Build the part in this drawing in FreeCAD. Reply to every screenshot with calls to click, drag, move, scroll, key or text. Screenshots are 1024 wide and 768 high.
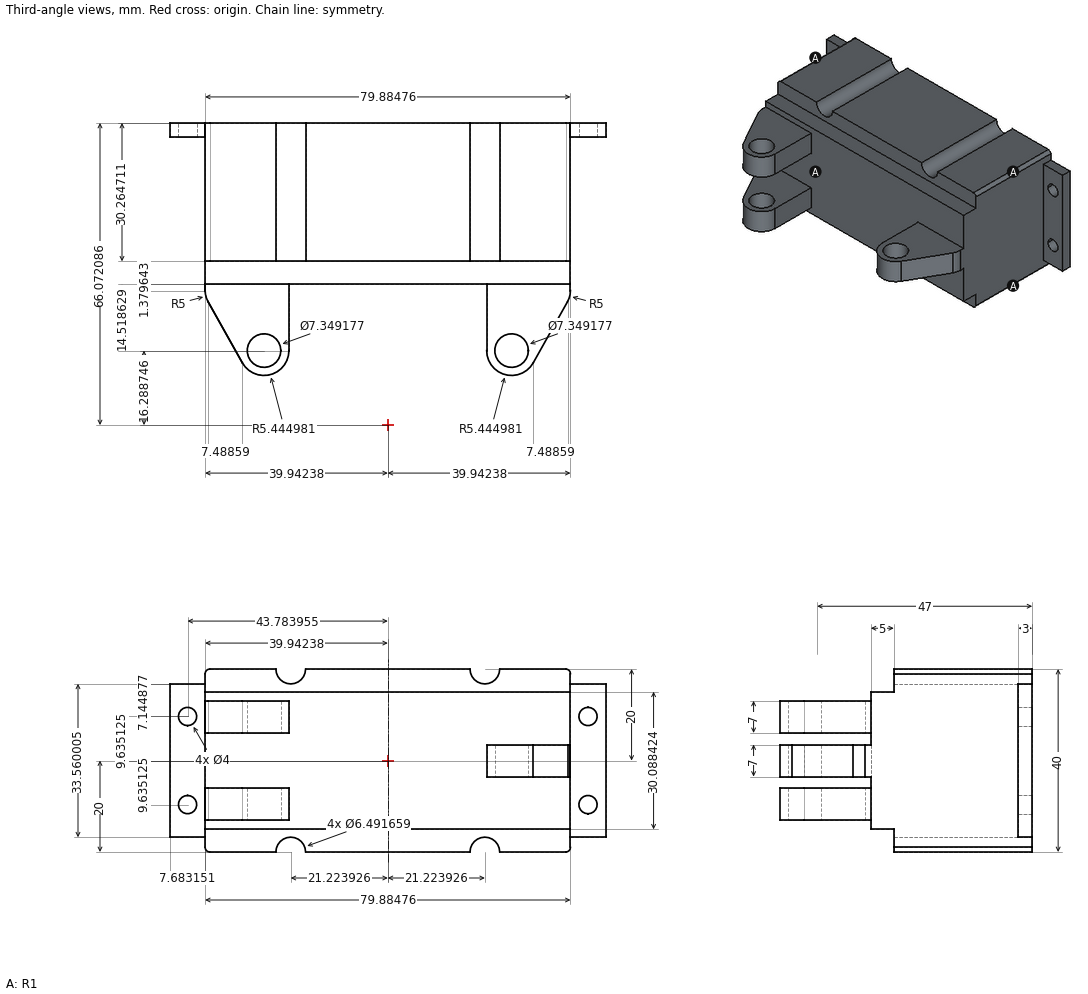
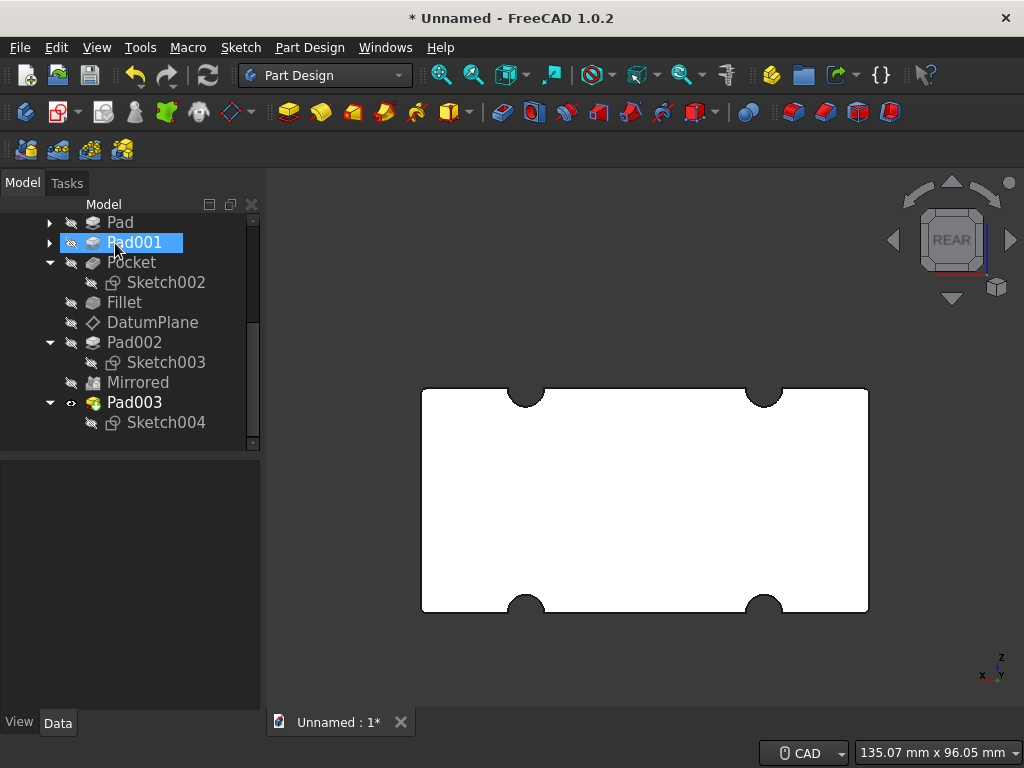
click(645, 500)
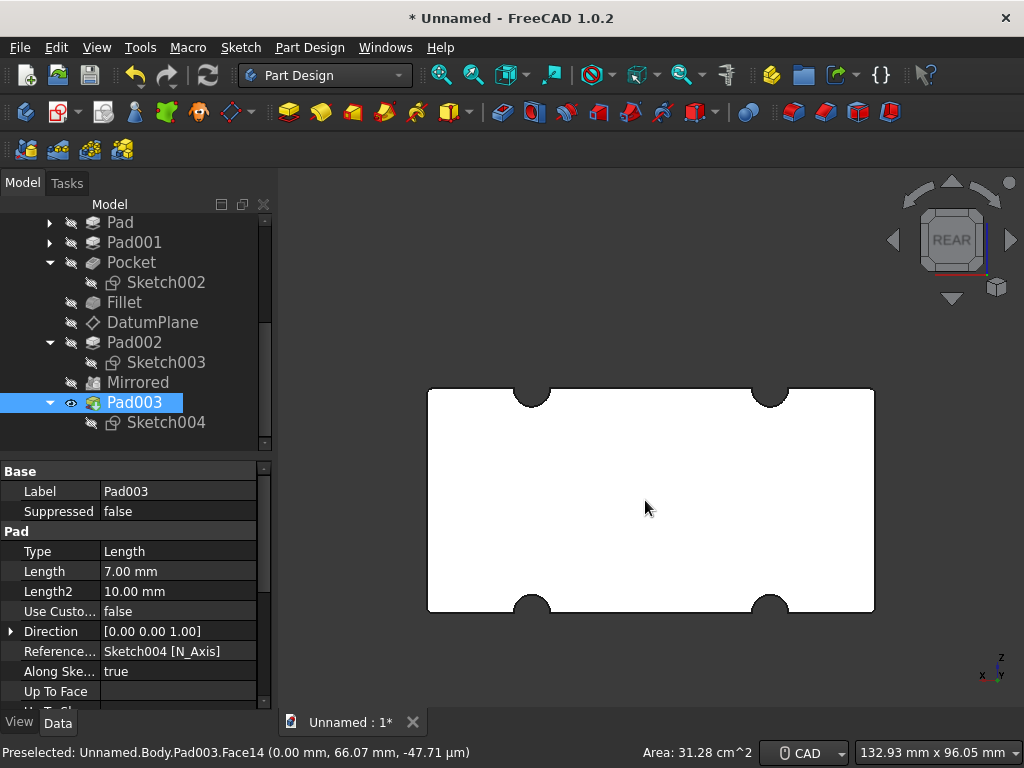
click(58, 112)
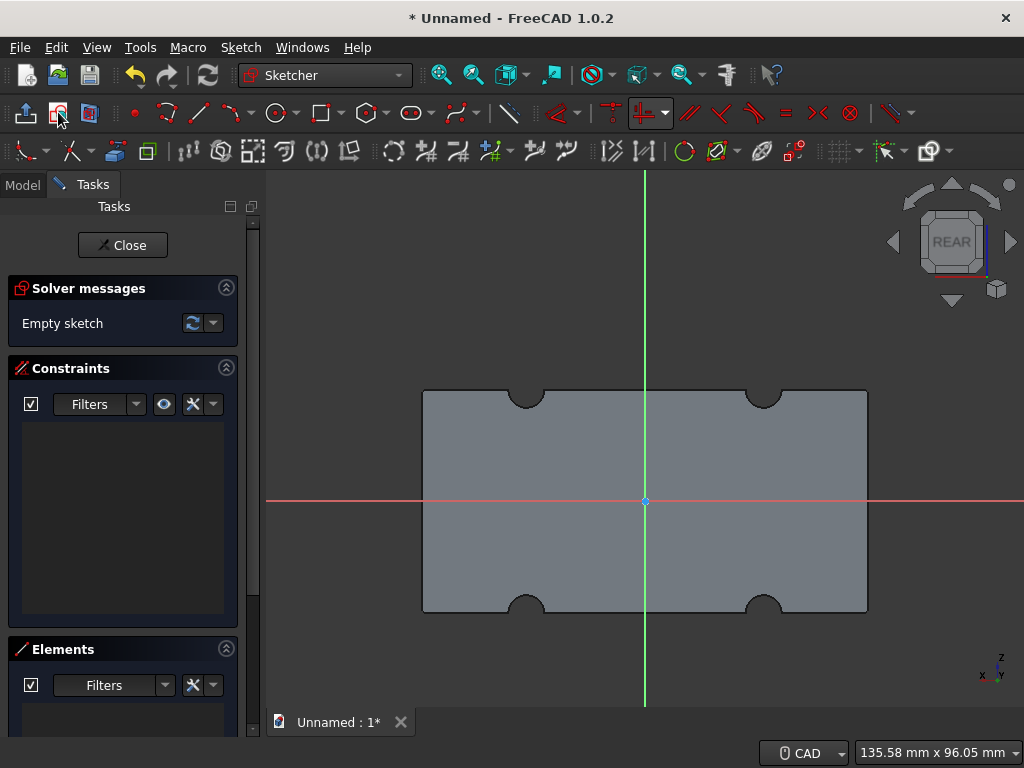
scroll(294, 198, down, 1)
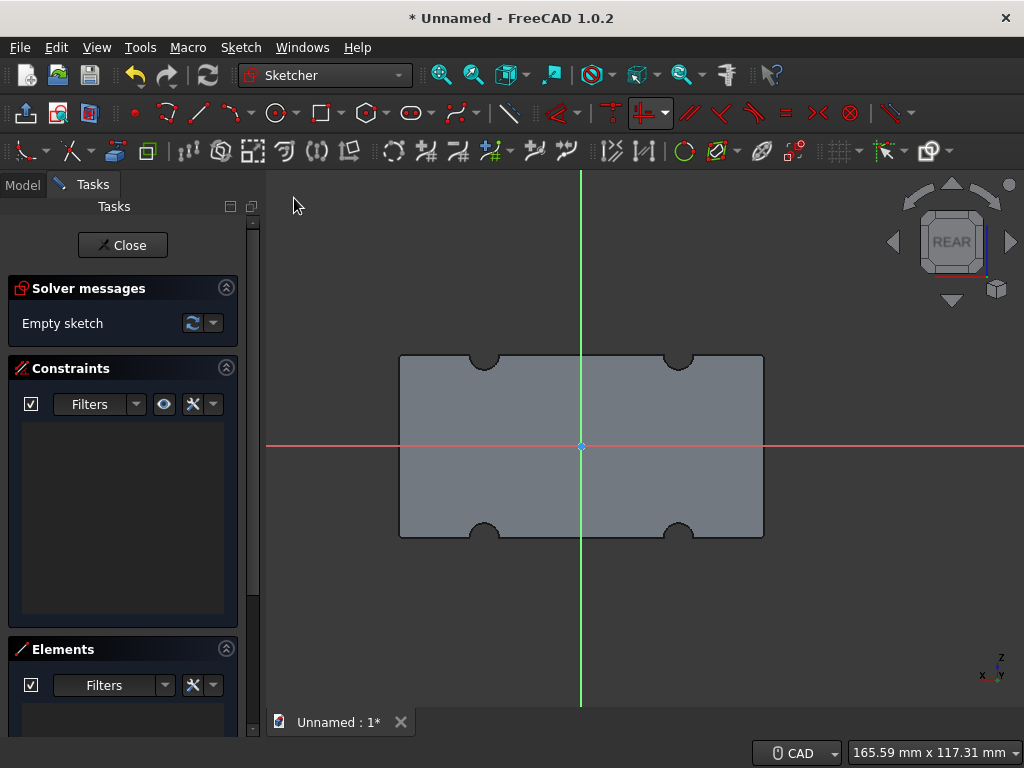
click(322, 114)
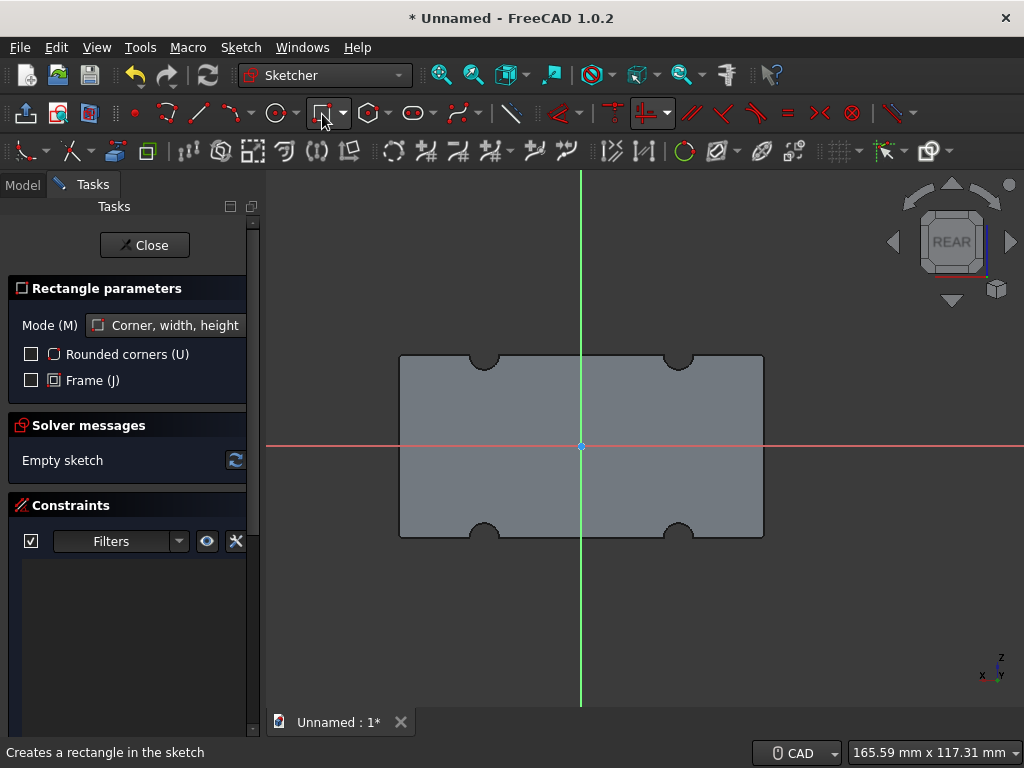
click(764, 370)
click(799, 523)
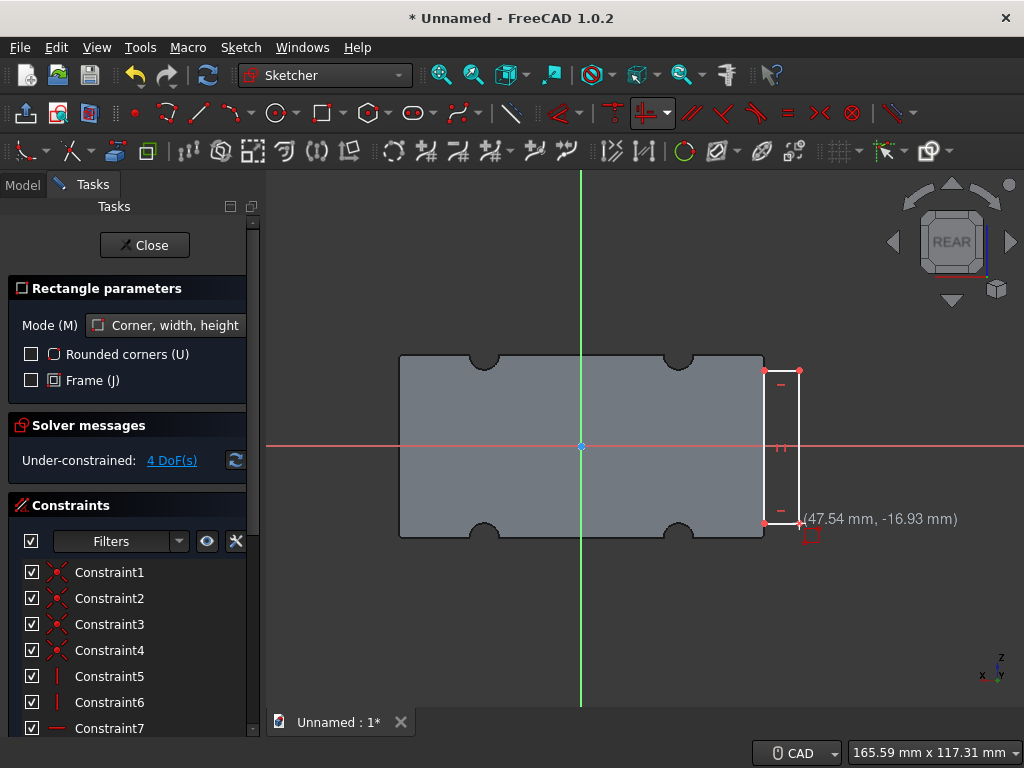
click(363, 370)
click(399, 523)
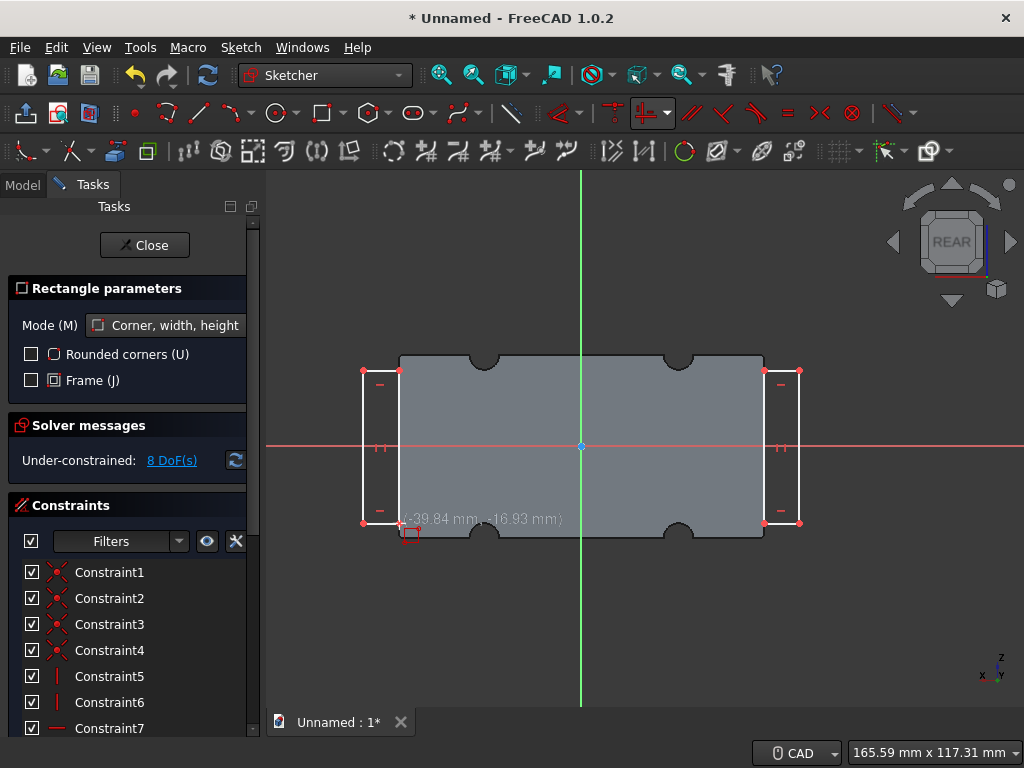
key(g)
key(c)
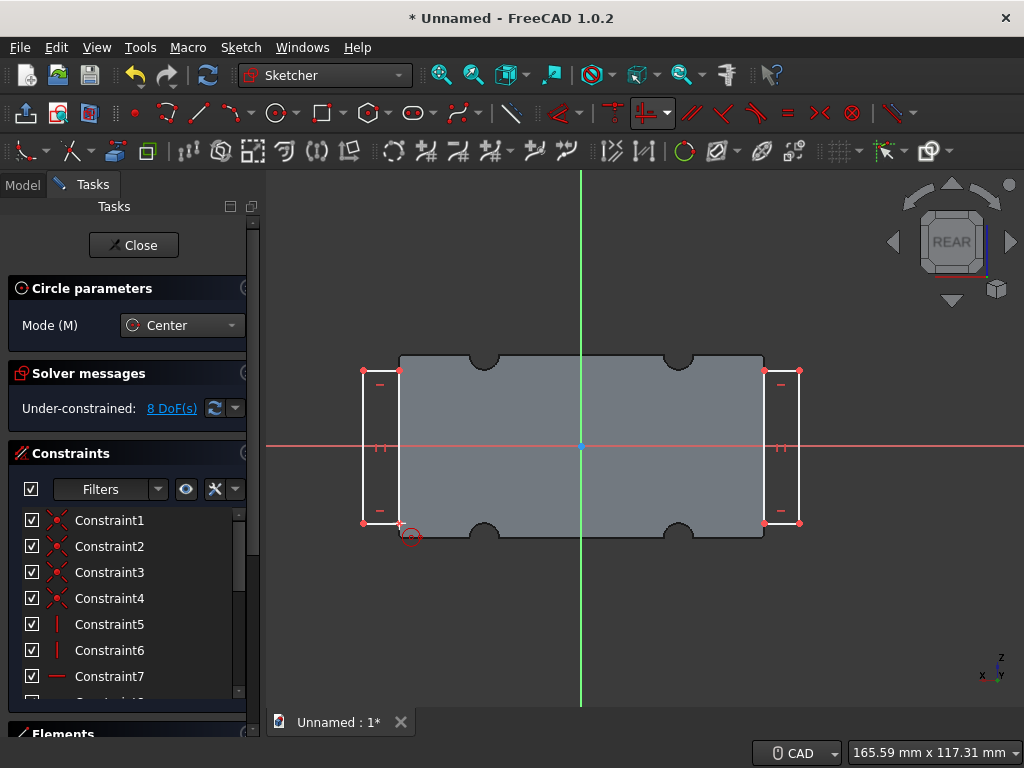
scroll(782, 402, up, 5)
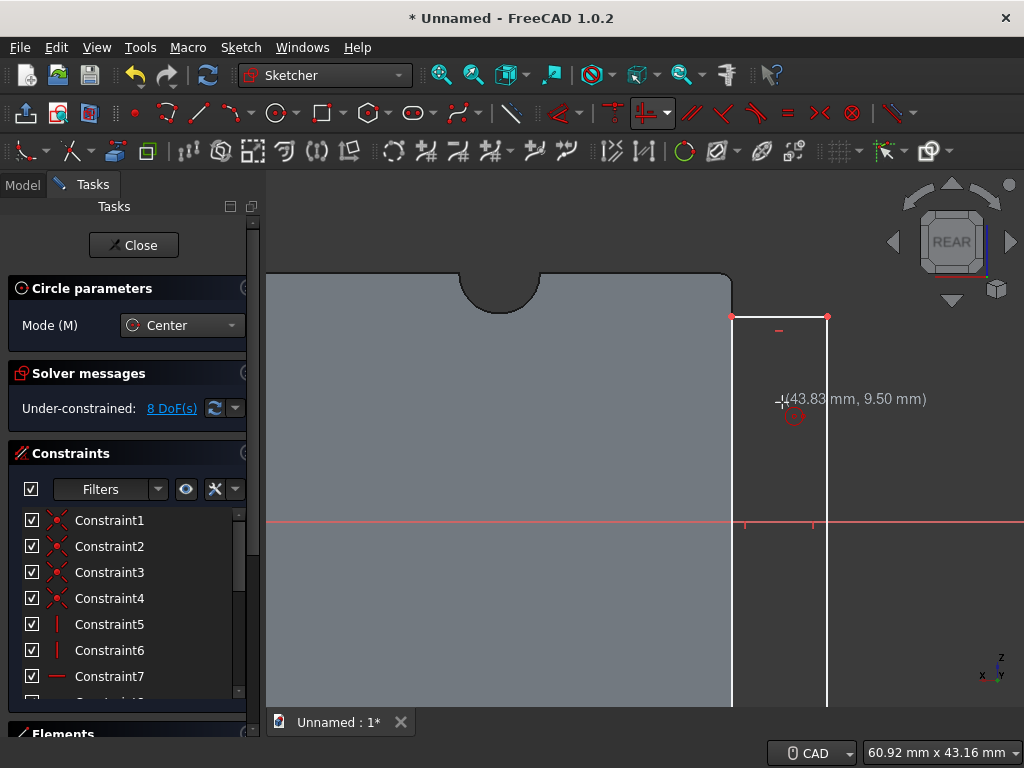
click(780, 402)
click(798, 385)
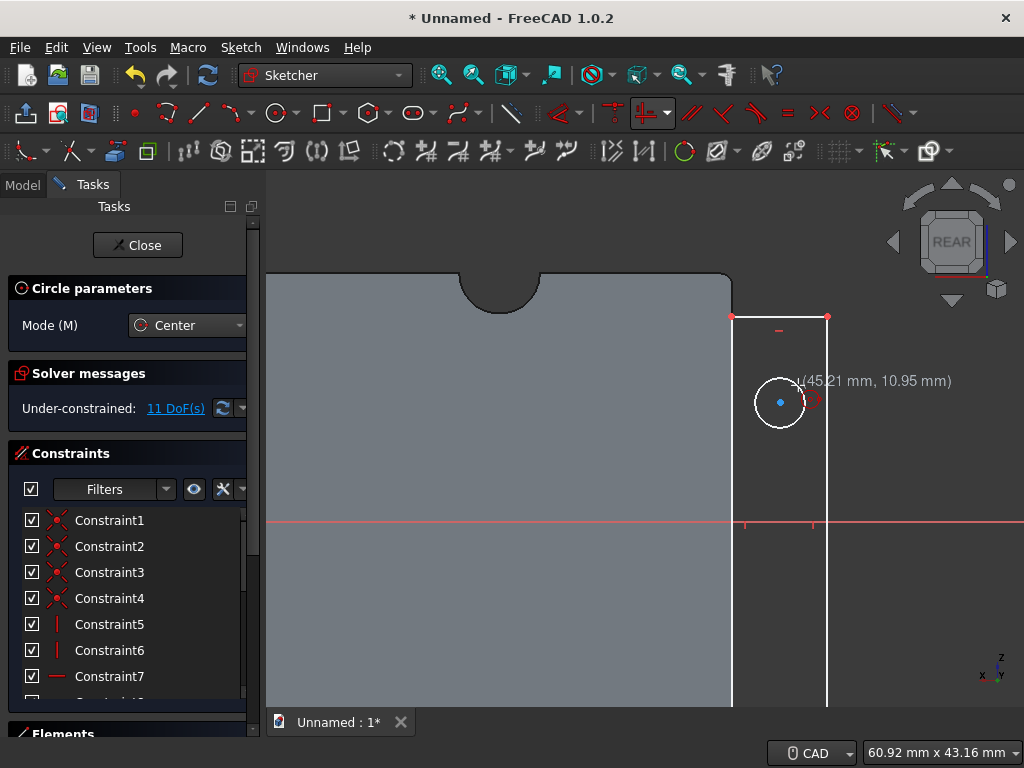
click(780, 642)
click(798, 624)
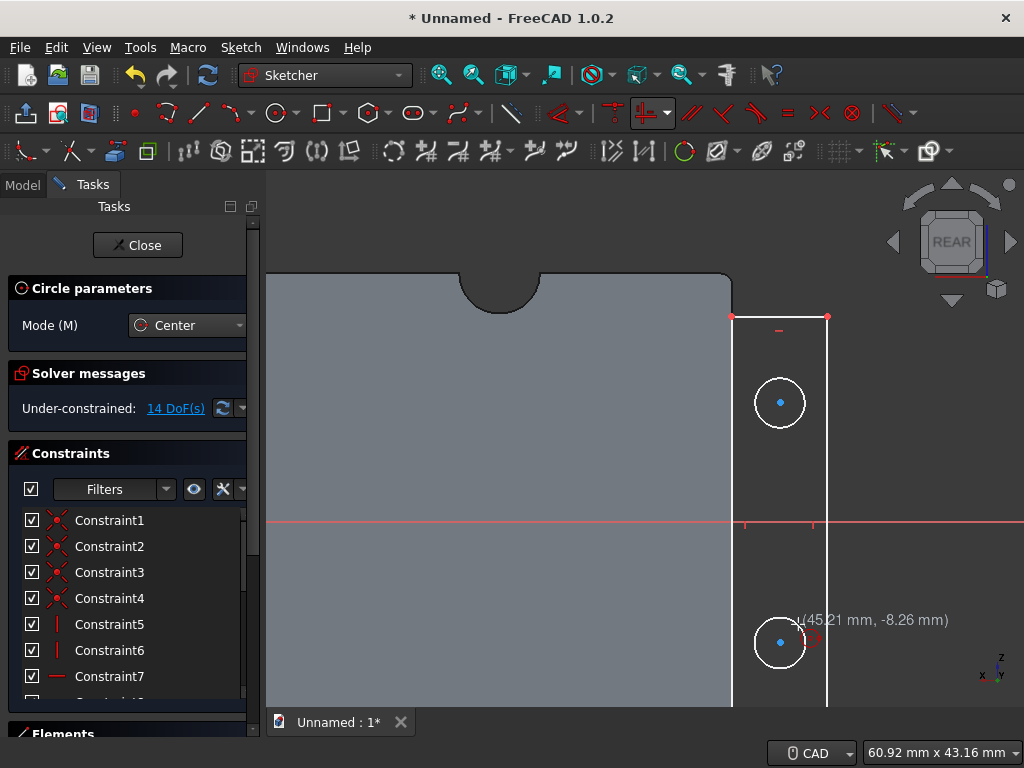
scroll(775, 390, down, 5)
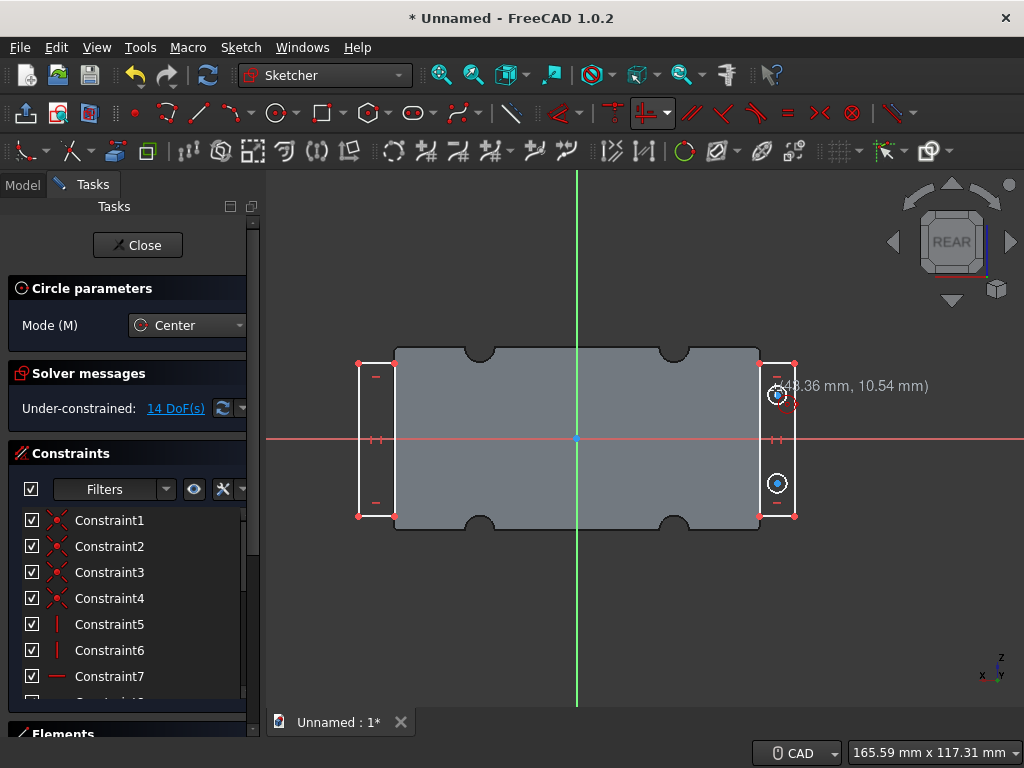
scroll(377, 395, up, 5)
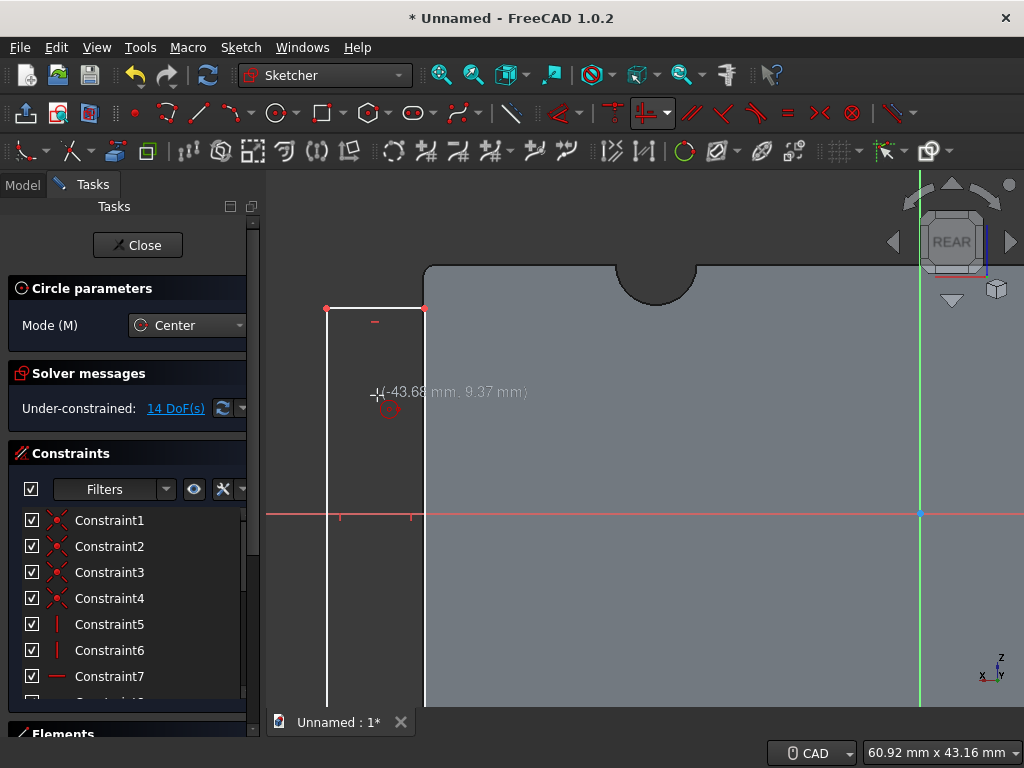
click(375, 394)
click(393, 376)